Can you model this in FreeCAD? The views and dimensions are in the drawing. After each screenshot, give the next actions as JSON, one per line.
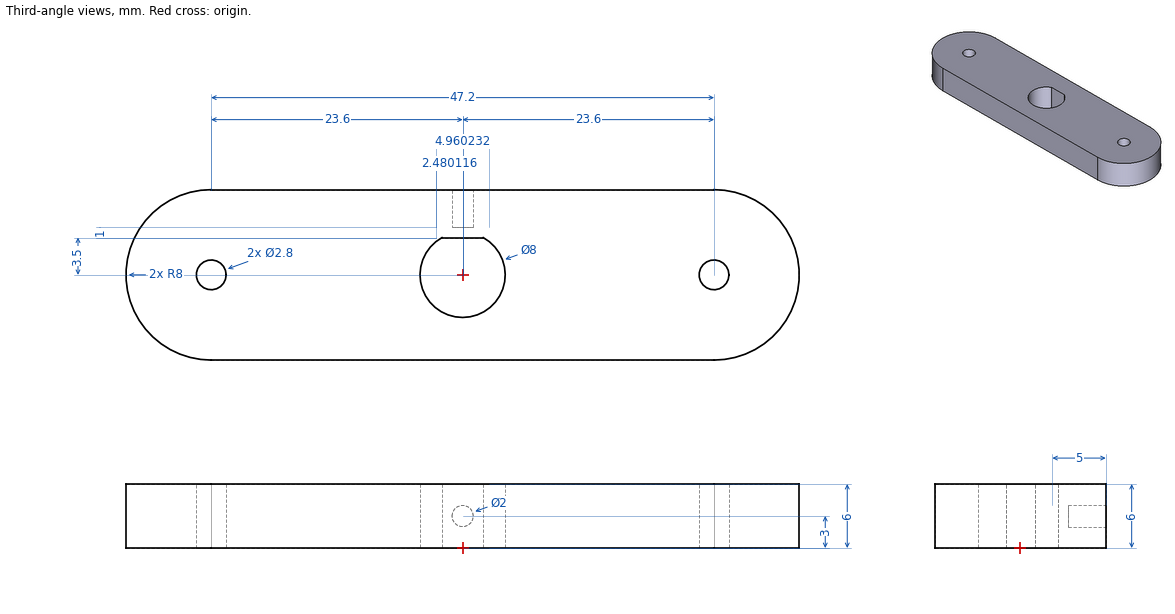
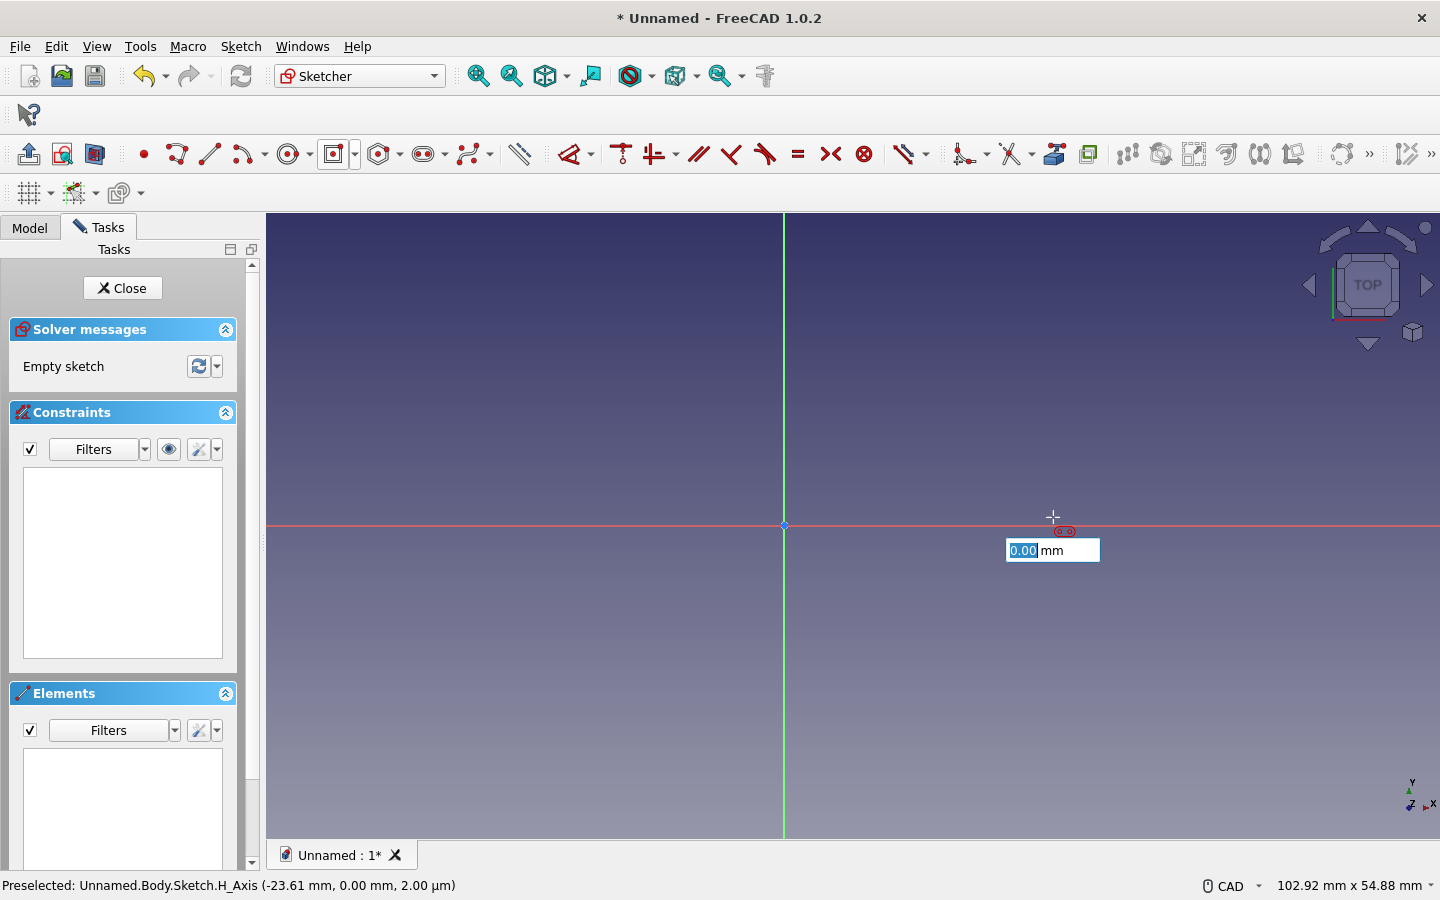
{"action": "left_click", "coordinate": [865, 434]}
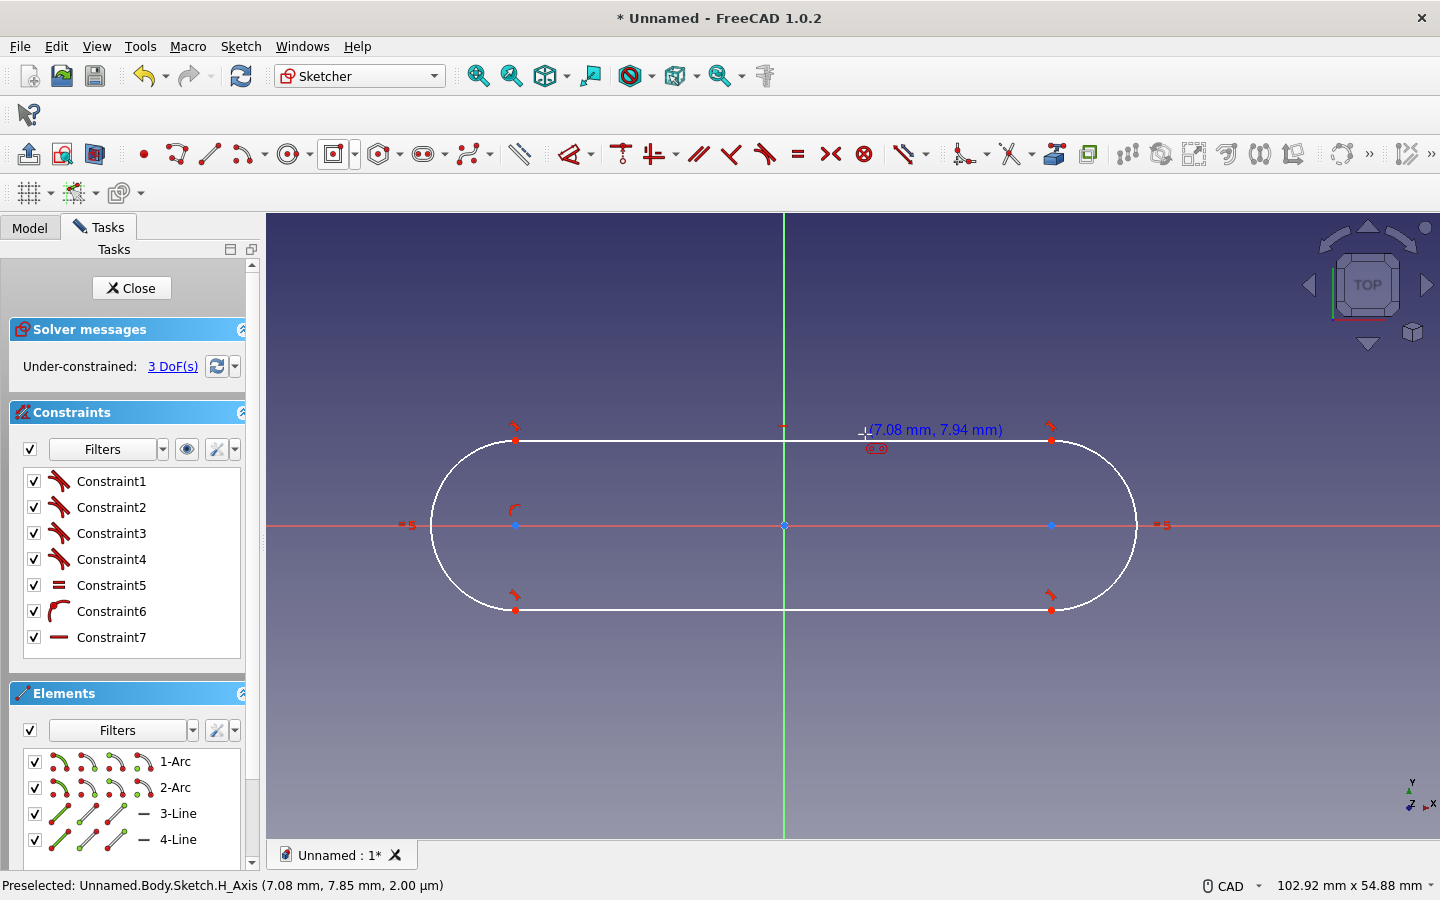
{"action": "left_click", "coordinate": [288, 154]}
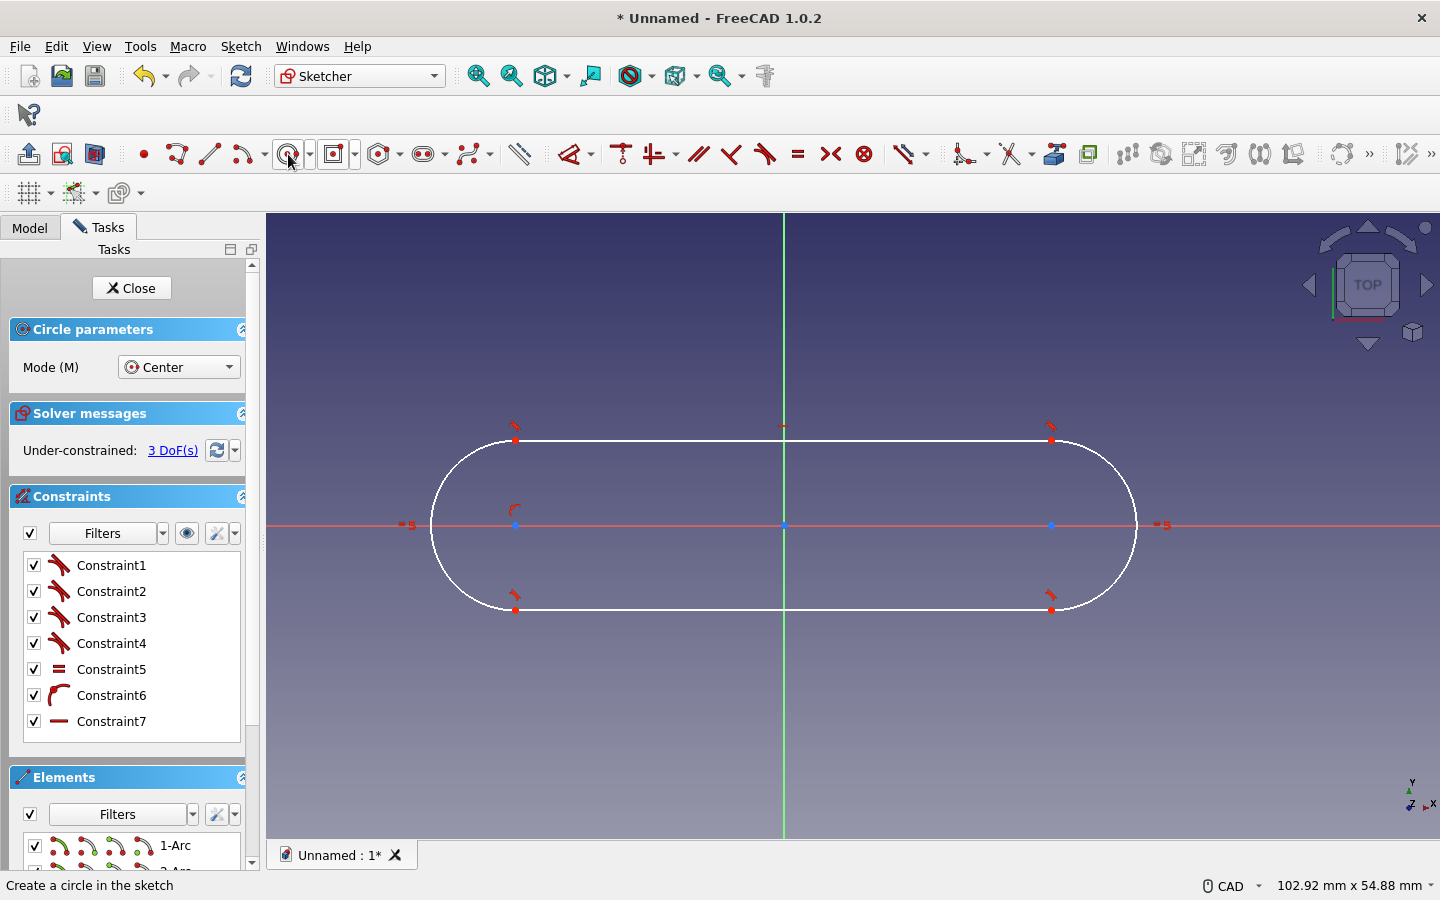
{"action": "left_click", "coordinate": [784, 526]}
{"action": "left_click", "coordinate": [817, 493]}
{"action": "key", "text": "Escape"}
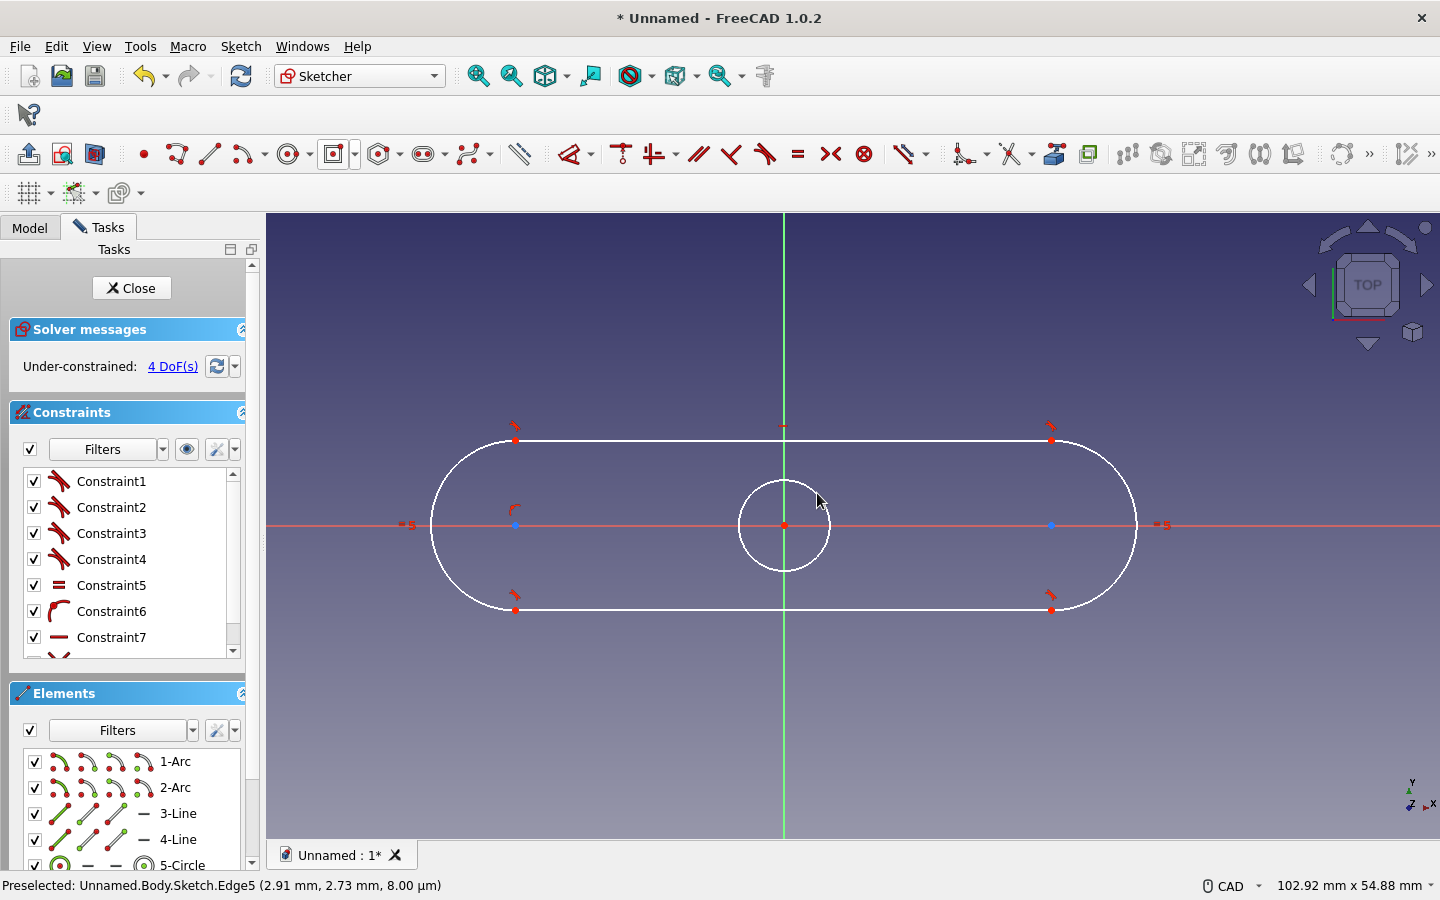
{"action": "left_click", "coordinate": [568, 154]}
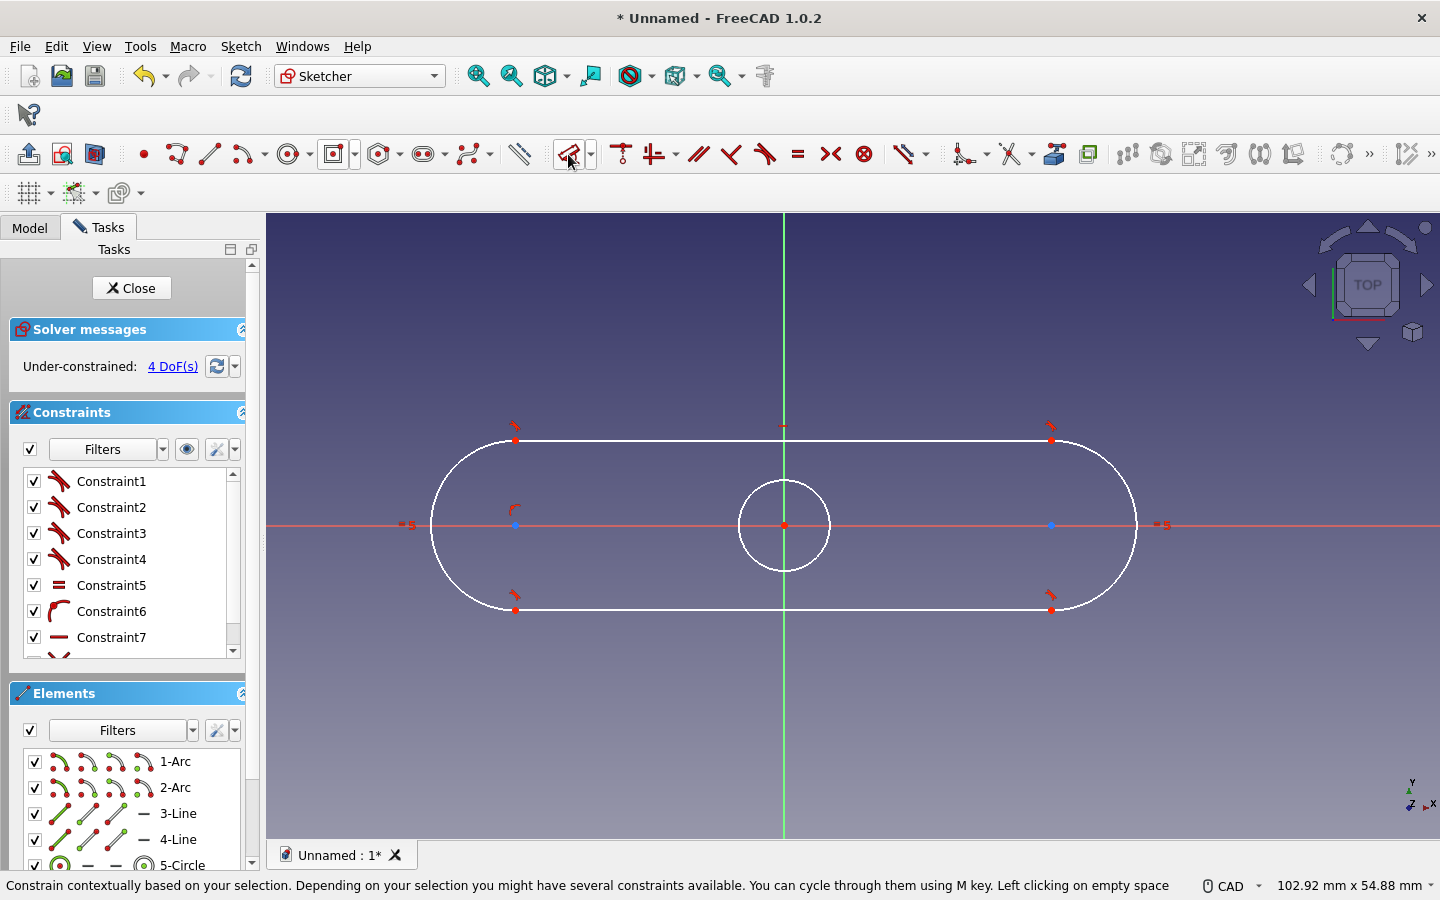
{"action": "left_click", "coordinate": [447, 476]}
{"action": "left_click", "coordinate": [421, 457]}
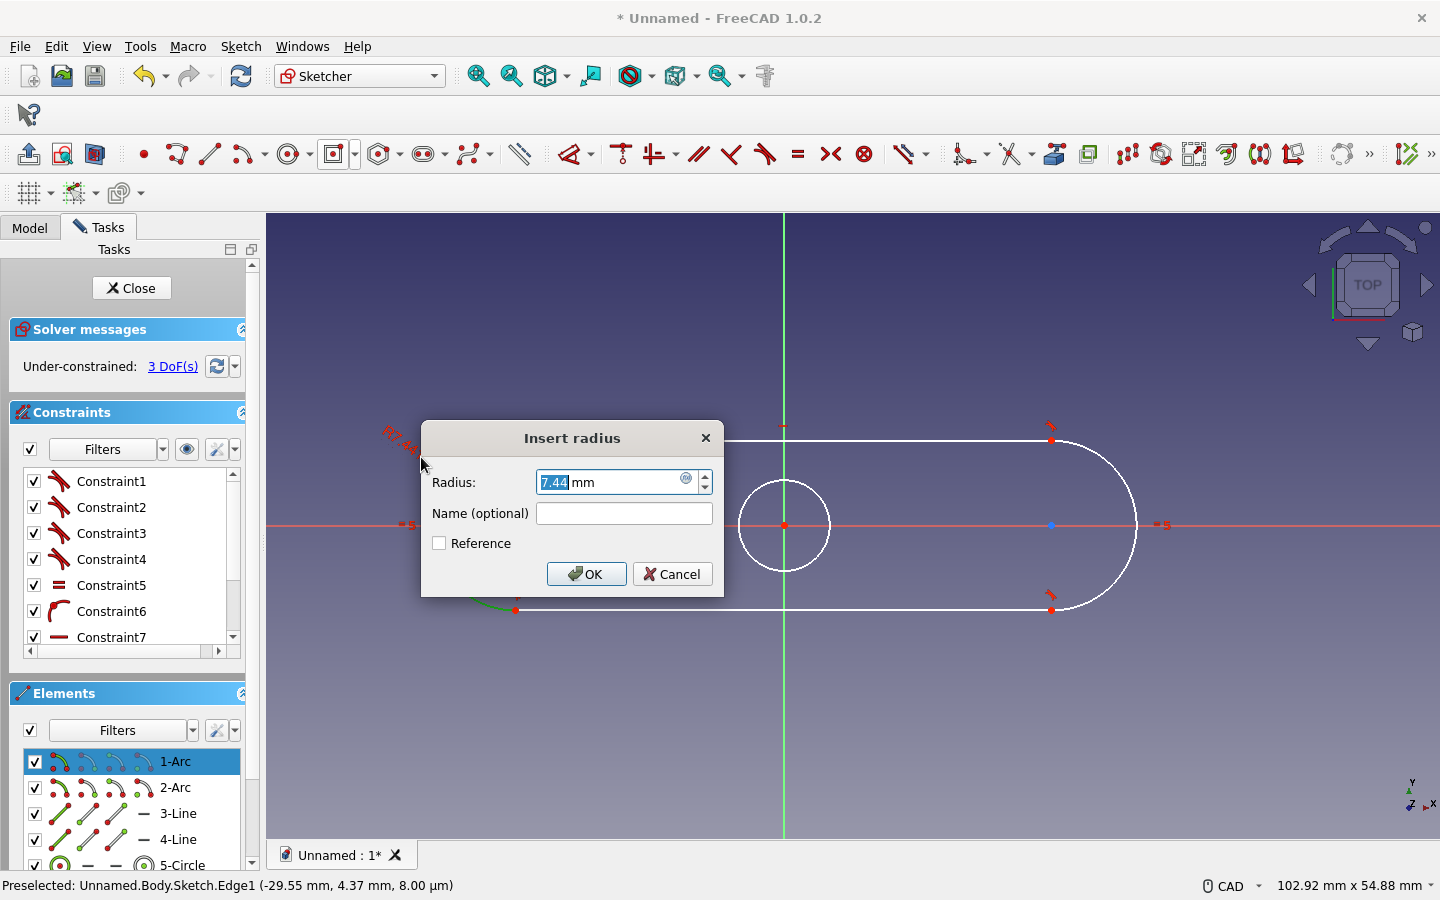
{"action": "type", "text": "8"}
{"action": "key", "text": "Return"}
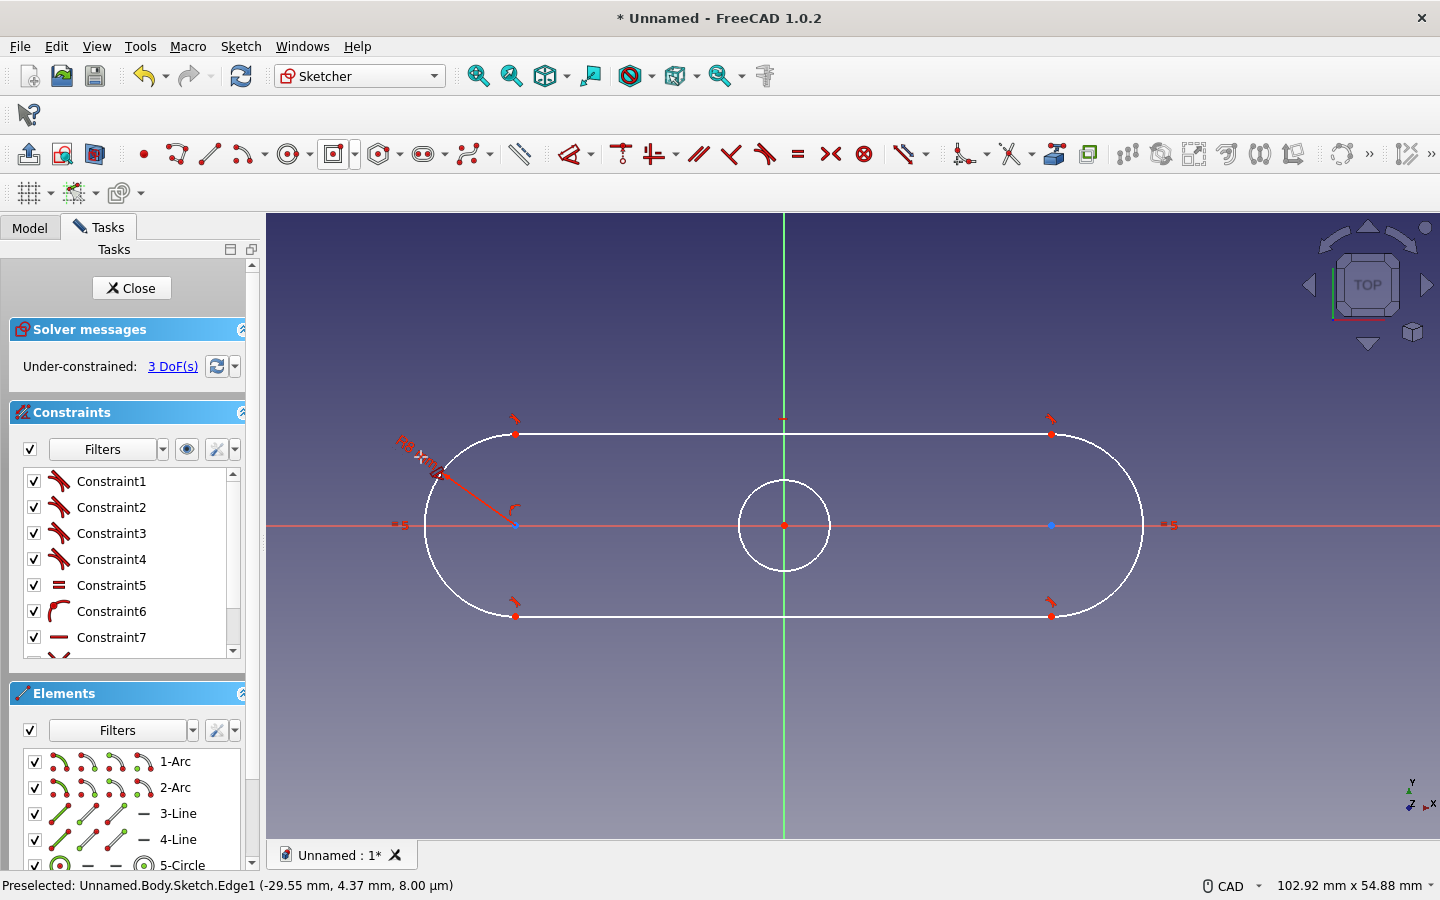
{"action": "left_click", "coordinate": [816, 493]}
{"action": "left_click", "coordinate": [838, 470]}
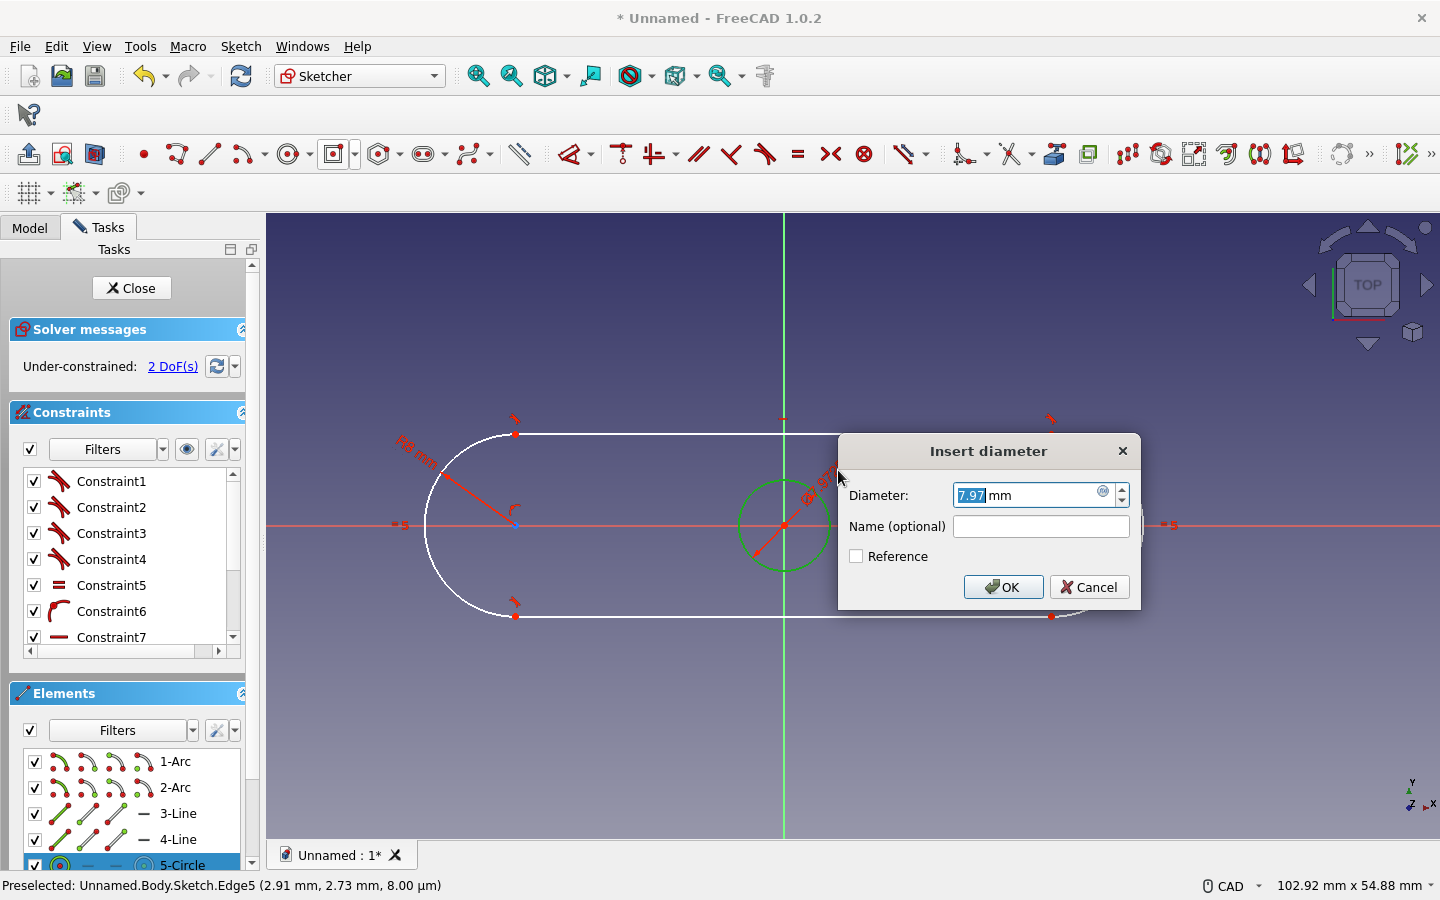
{"action": "type", "text": "8"}
{"action": "key", "text": "Return"}